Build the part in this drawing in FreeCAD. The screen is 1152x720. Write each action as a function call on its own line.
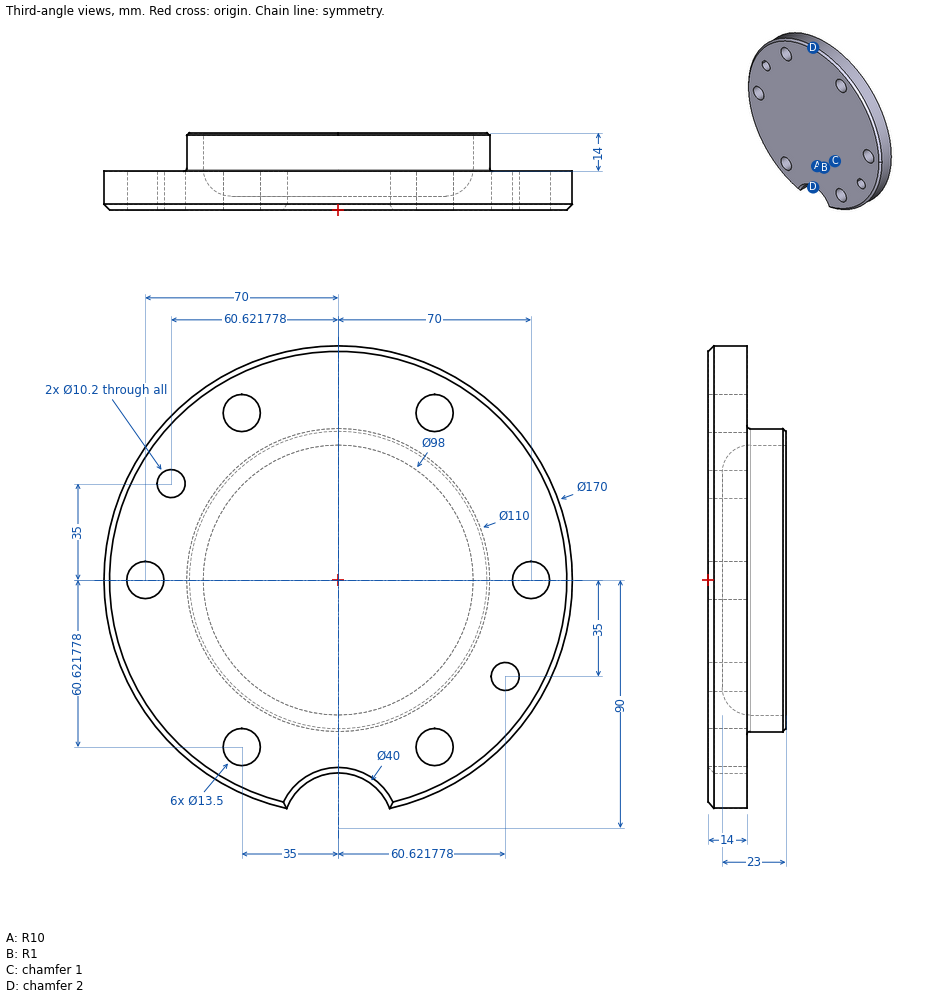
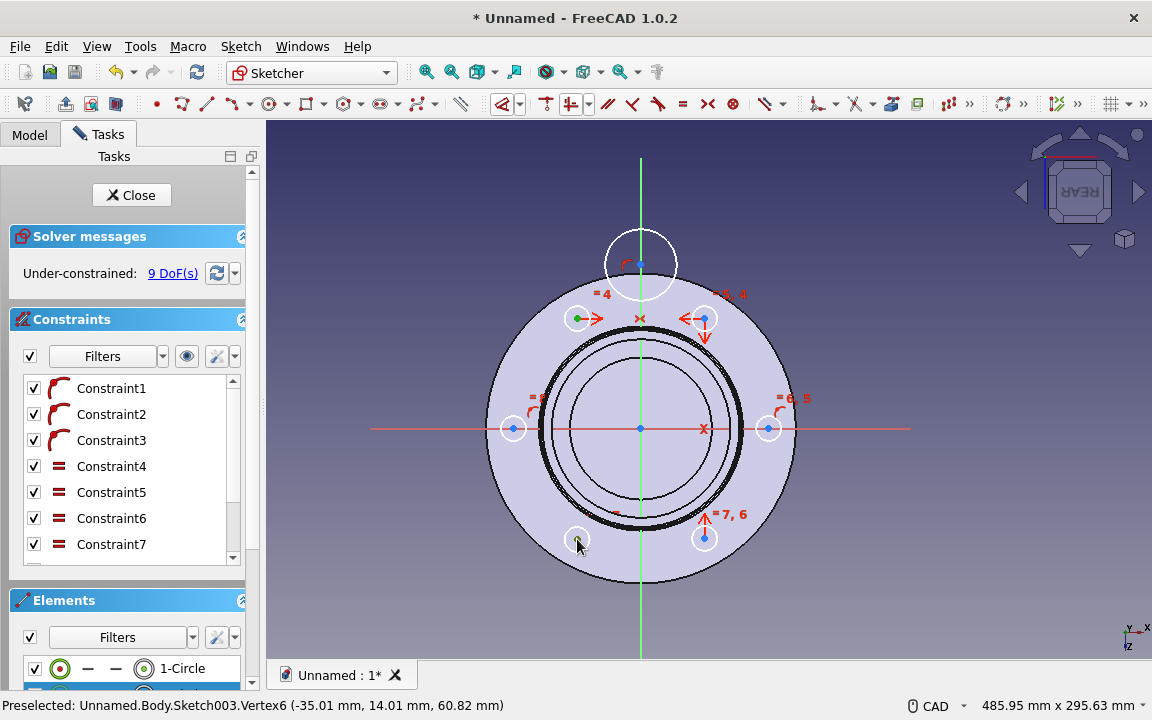
click(393, 429)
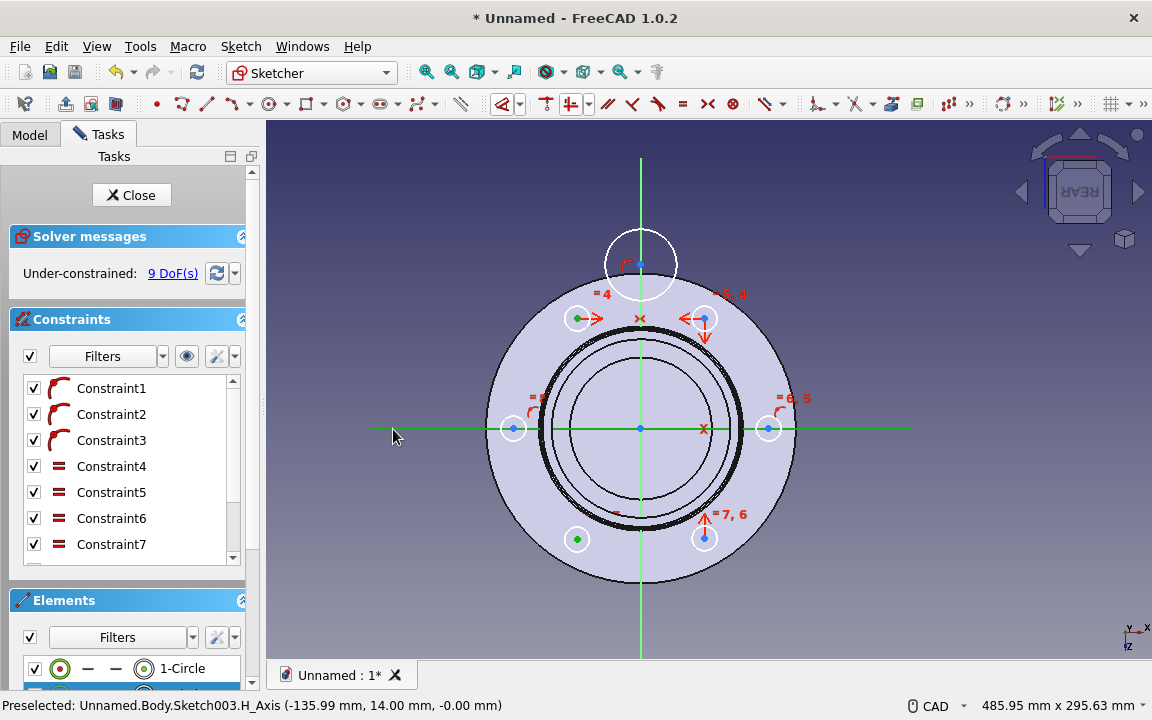
click(708, 104)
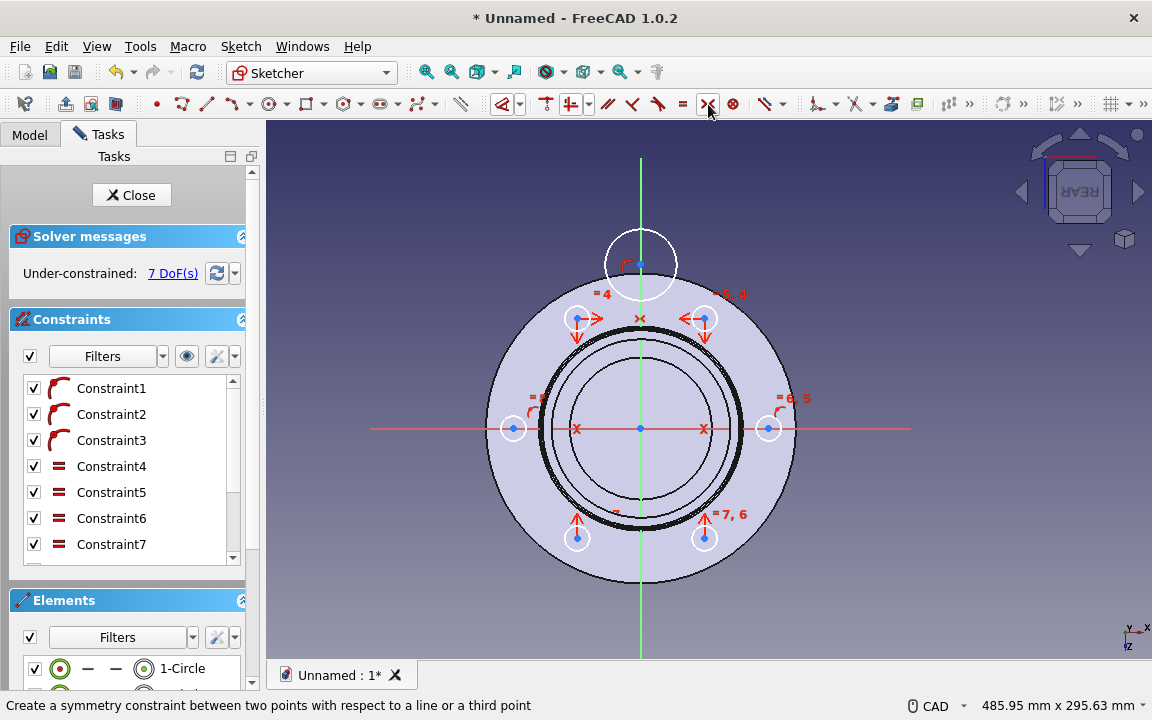
click(666, 240)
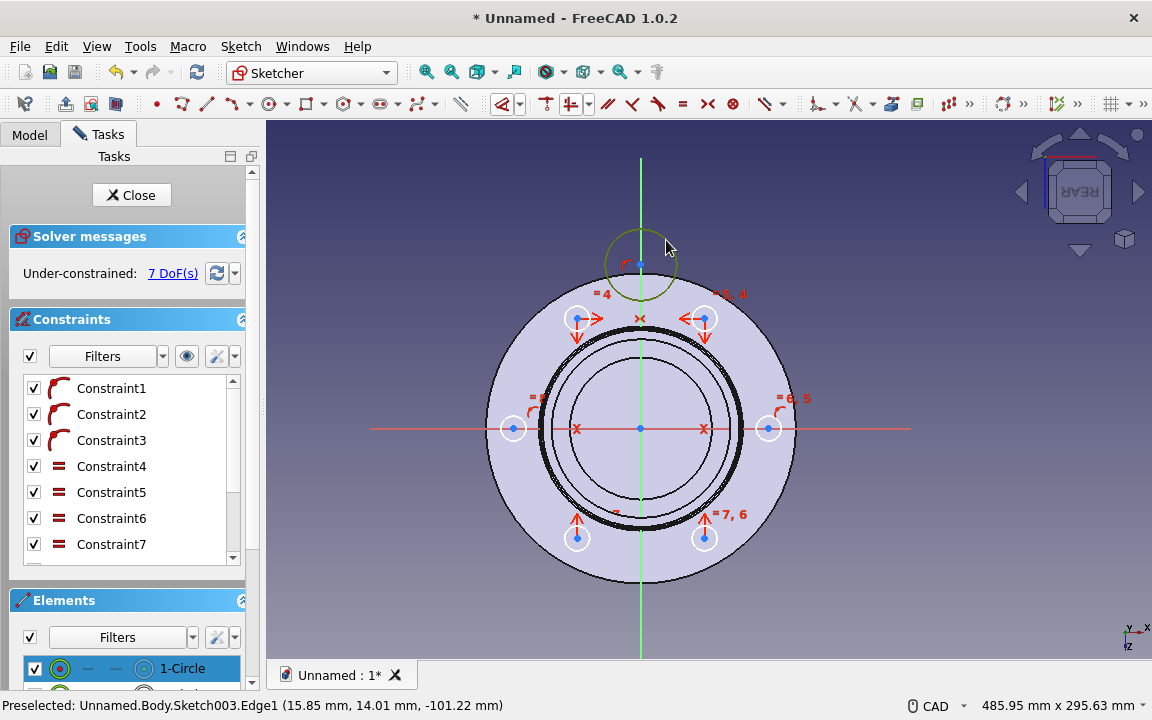
click(520, 104)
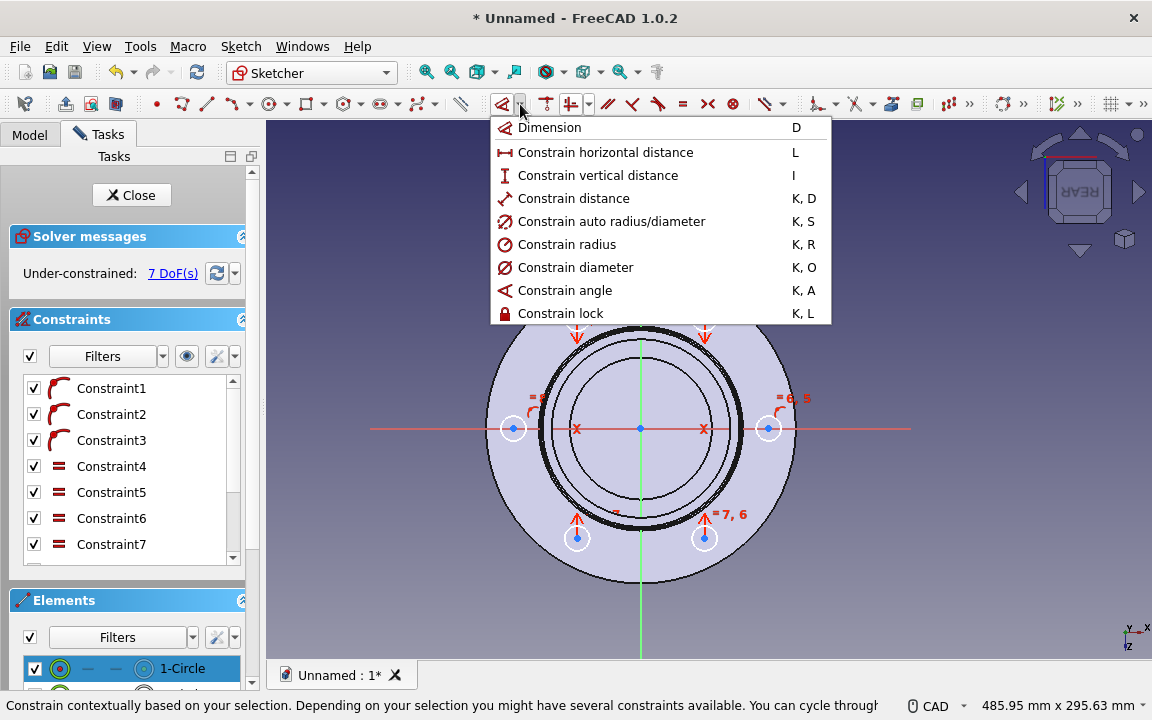
click(661, 268)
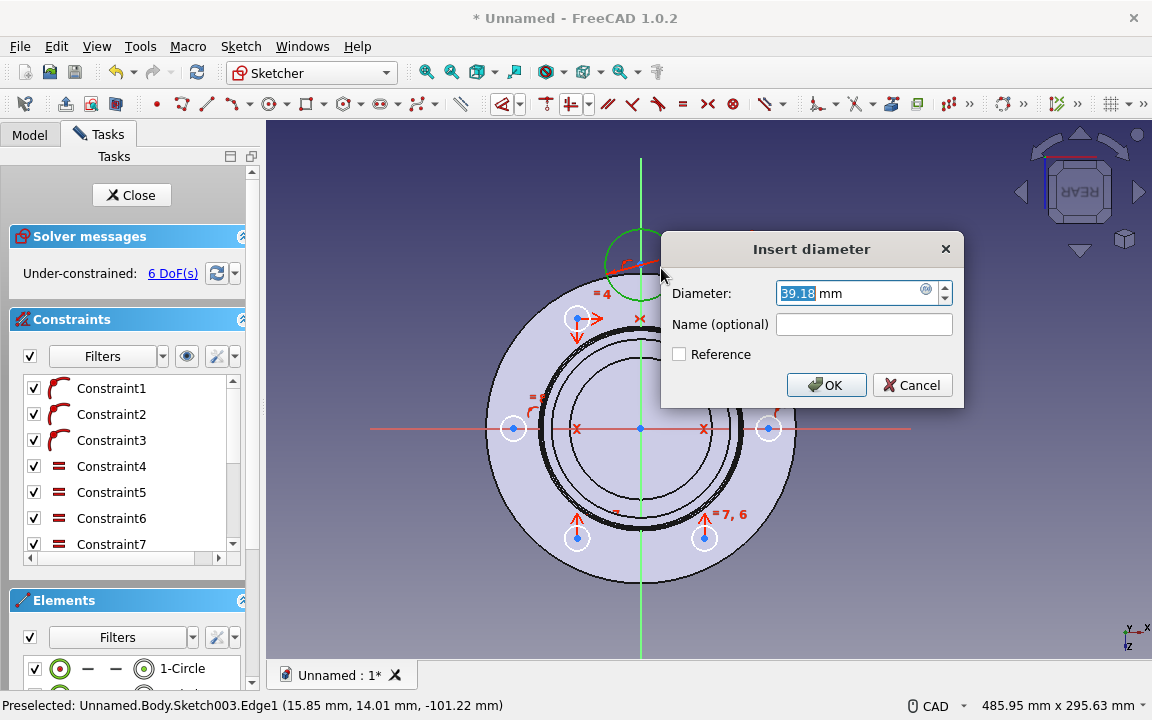
text(40)
key(Return)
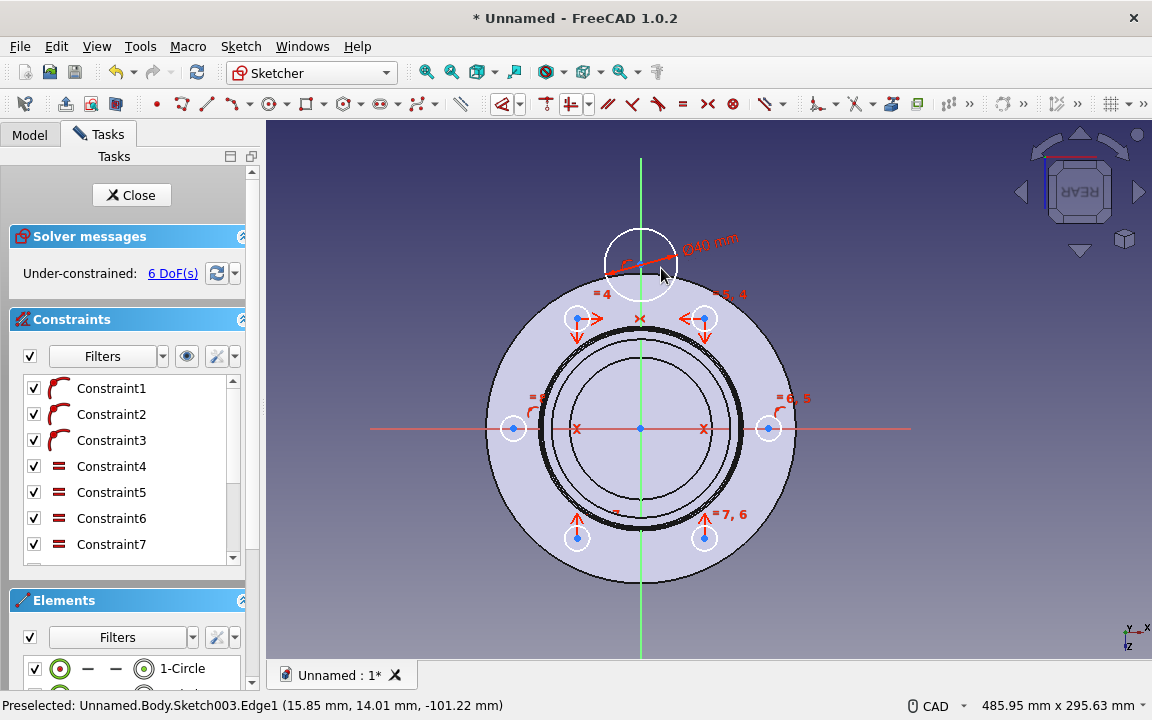
scroll(586, 310, up, 3)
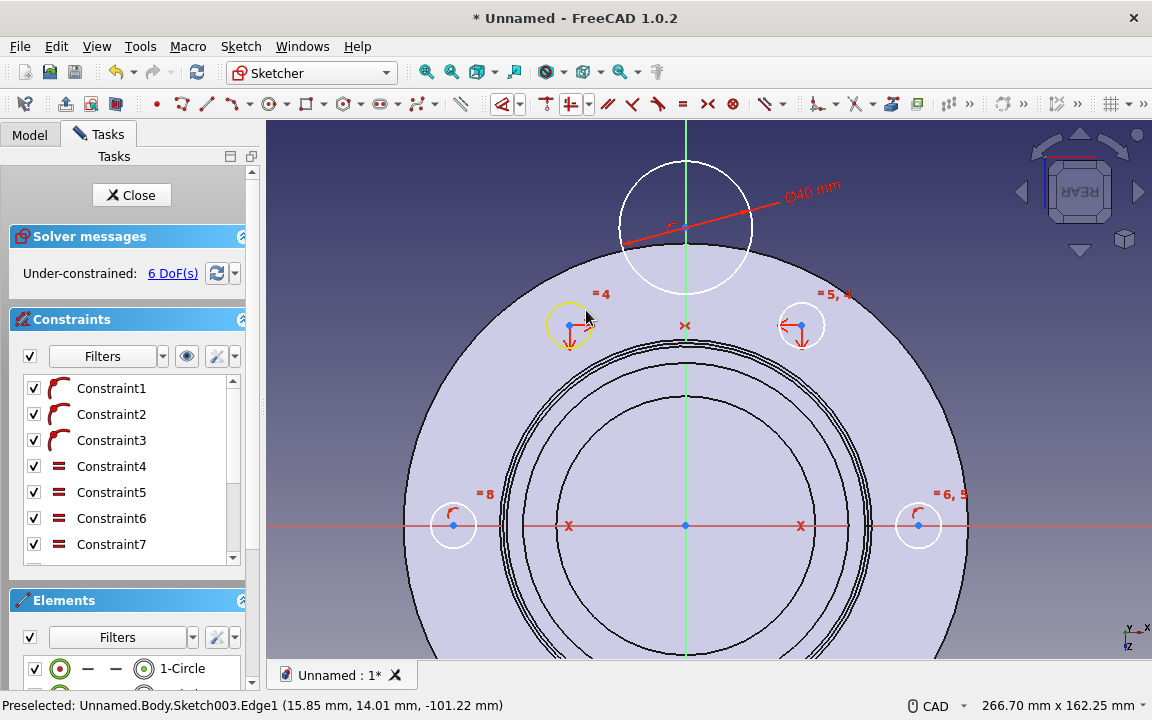
click(586, 309)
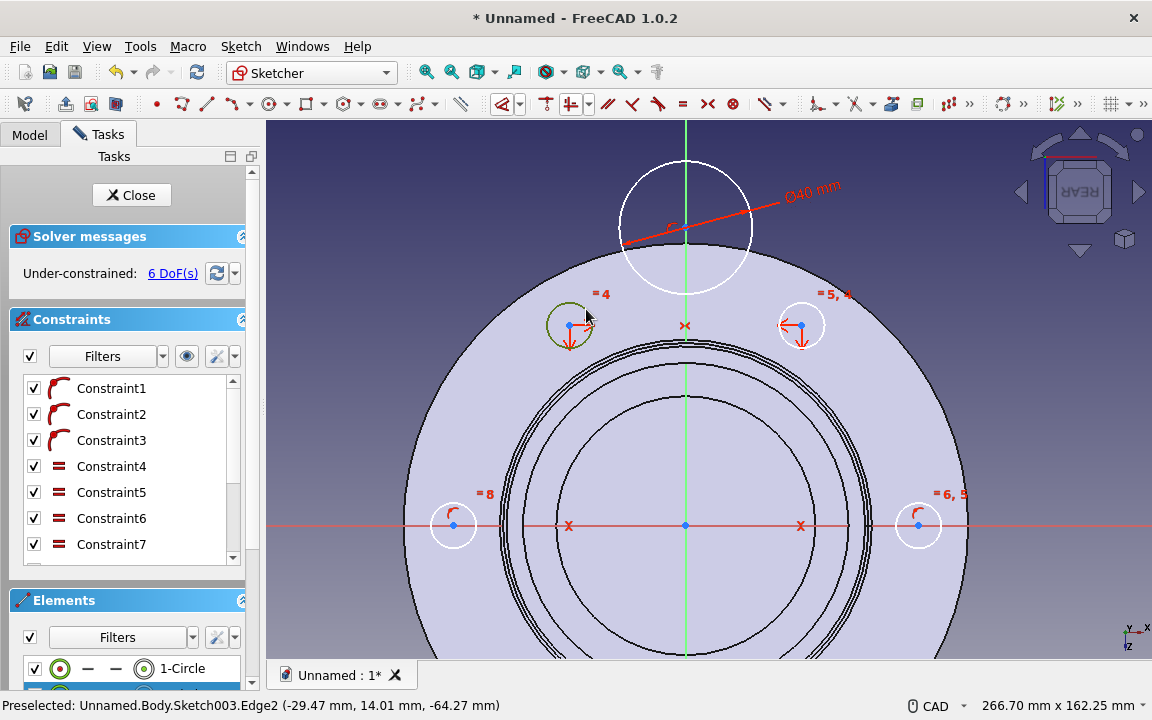
key(k)
key(o)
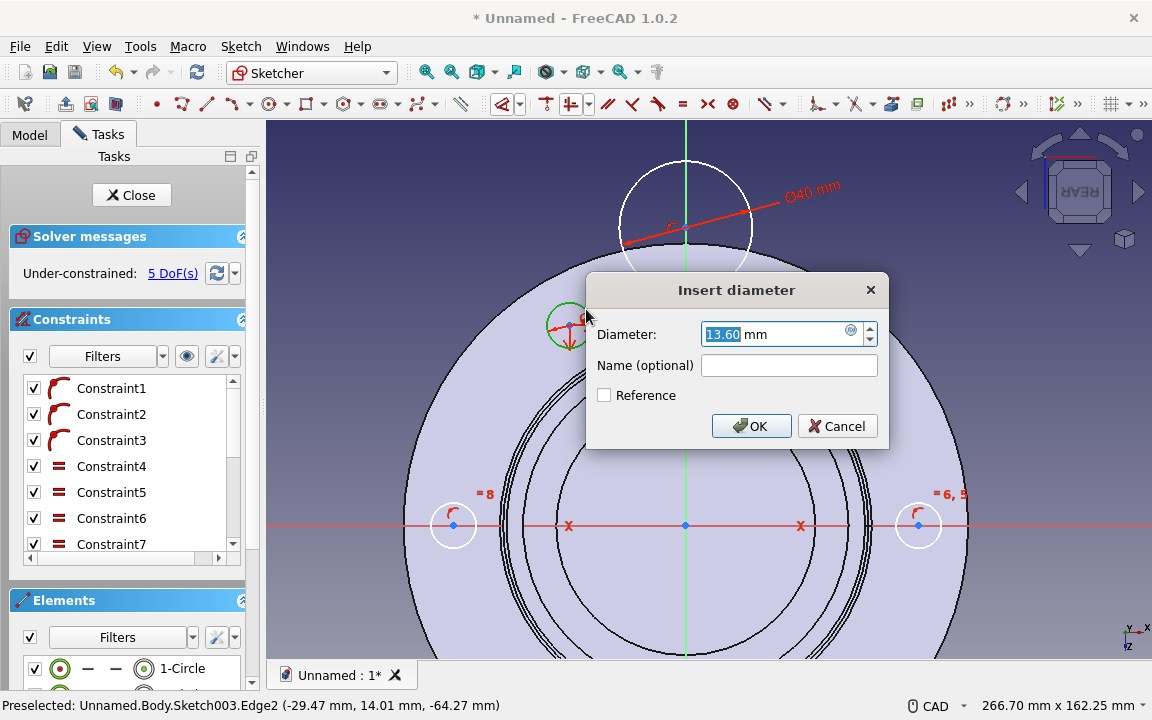
text(13.5)
key(Return)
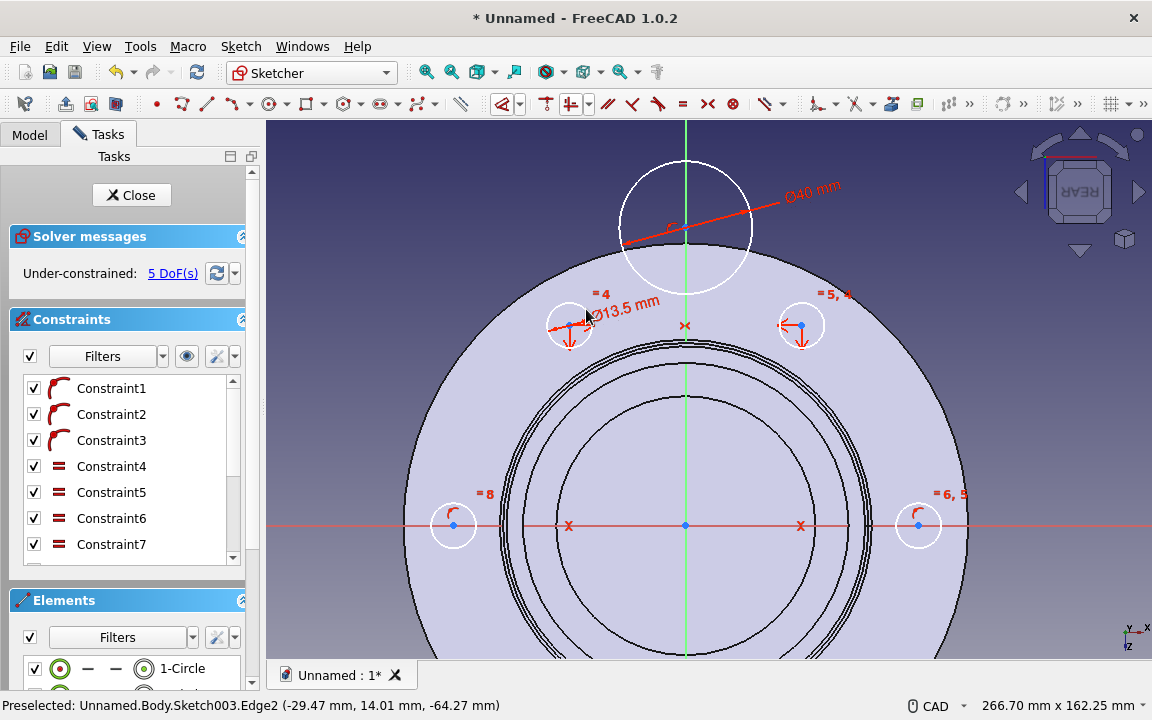
click(686, 228)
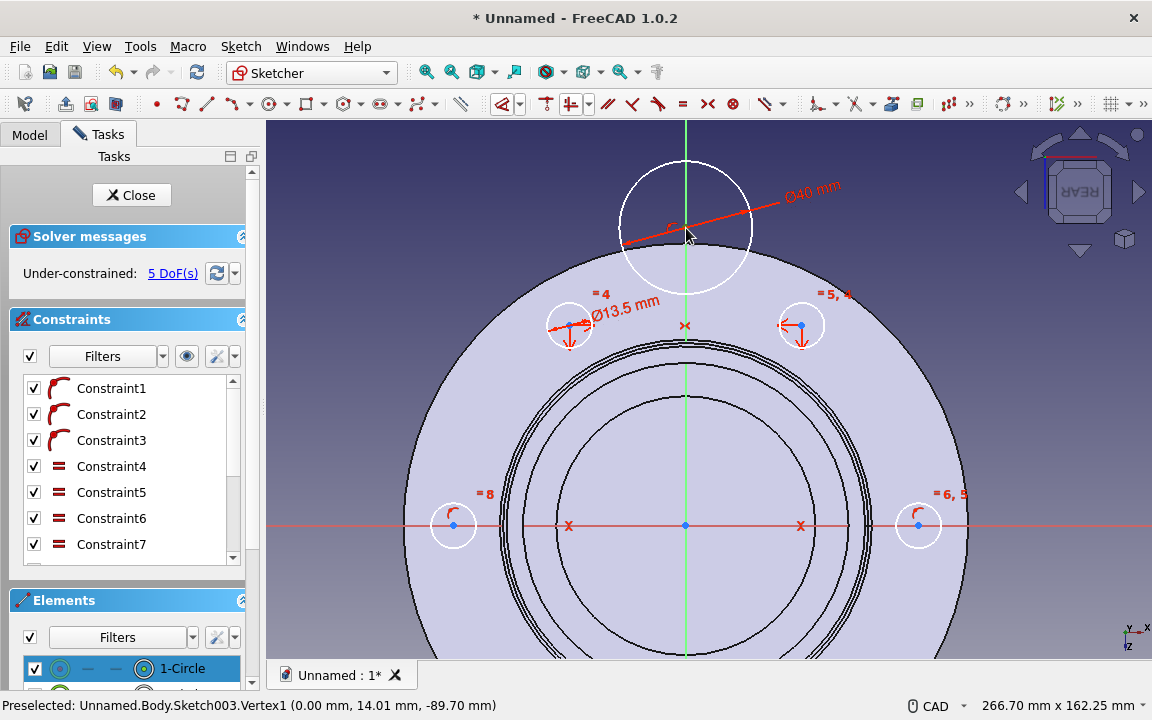
key(i)